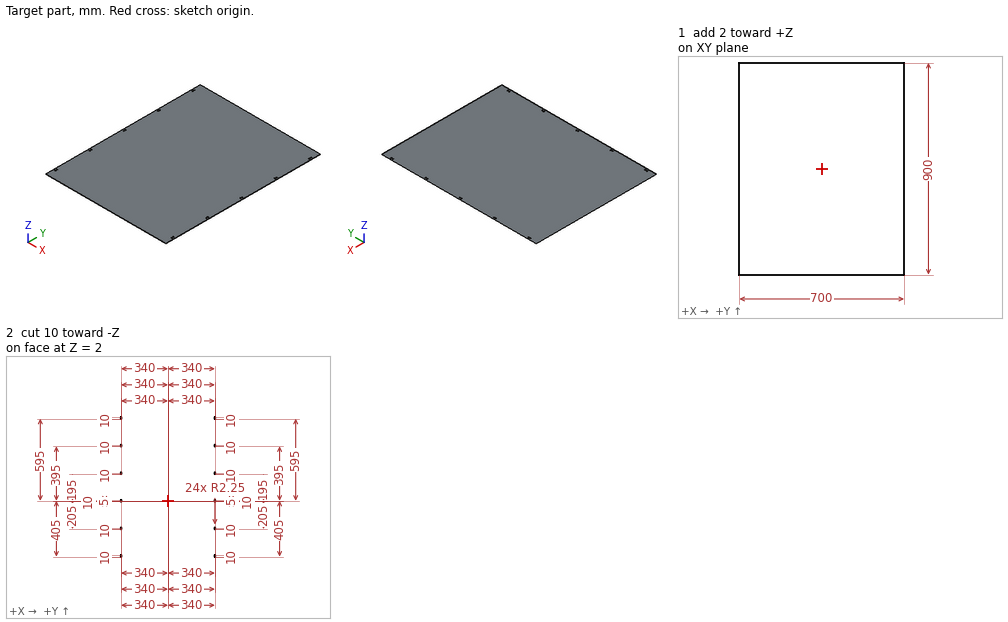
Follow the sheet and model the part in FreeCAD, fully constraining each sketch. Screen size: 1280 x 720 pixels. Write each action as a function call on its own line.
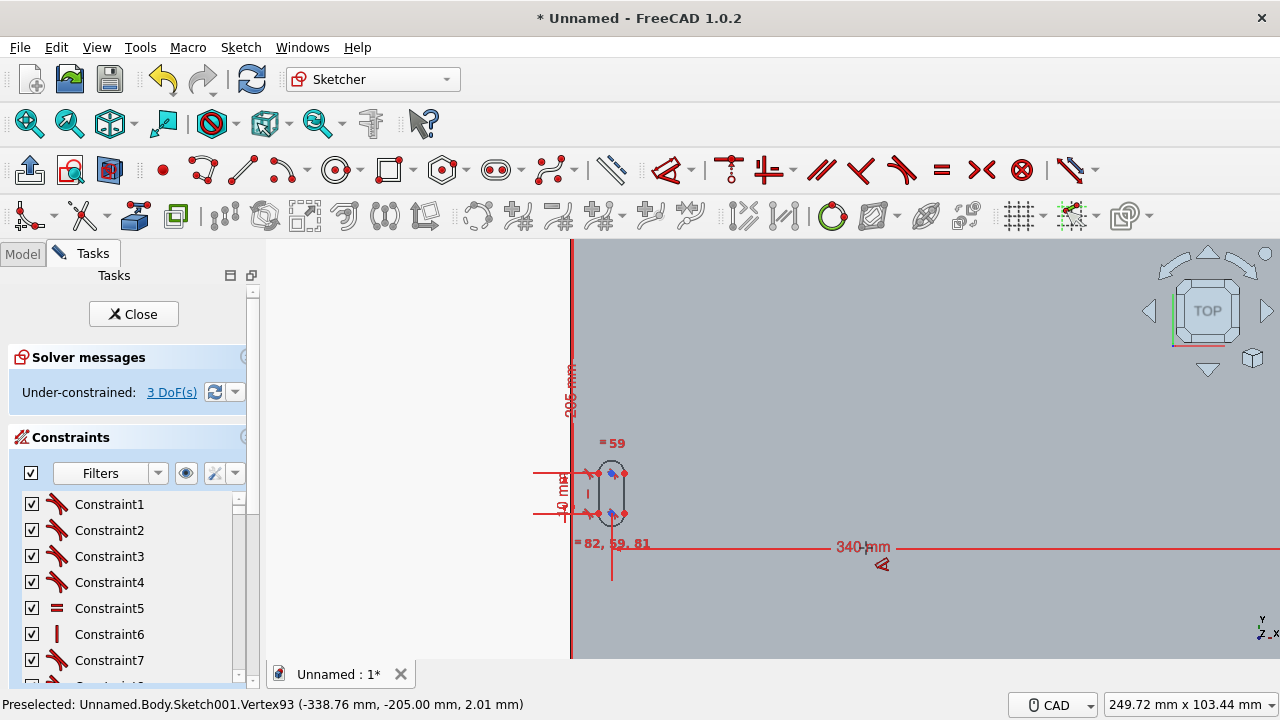
scroll(621, 525, down, 14)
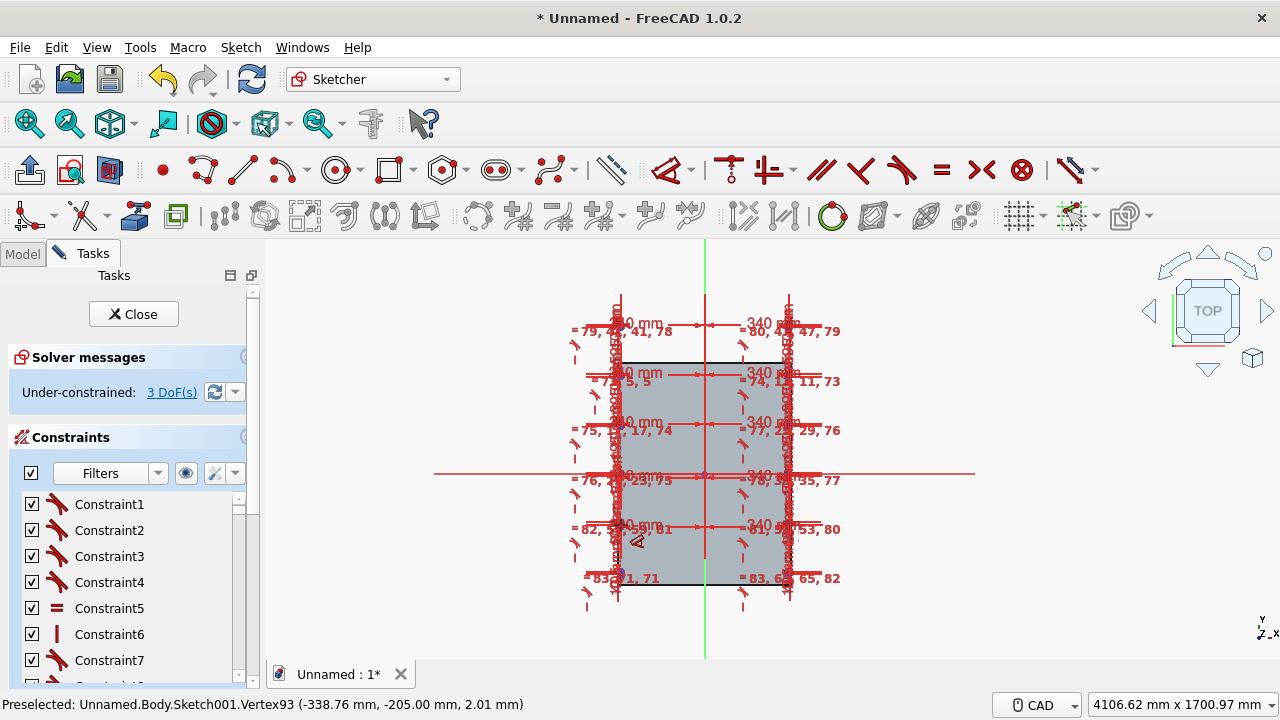
scroll(789, 574, up, 14)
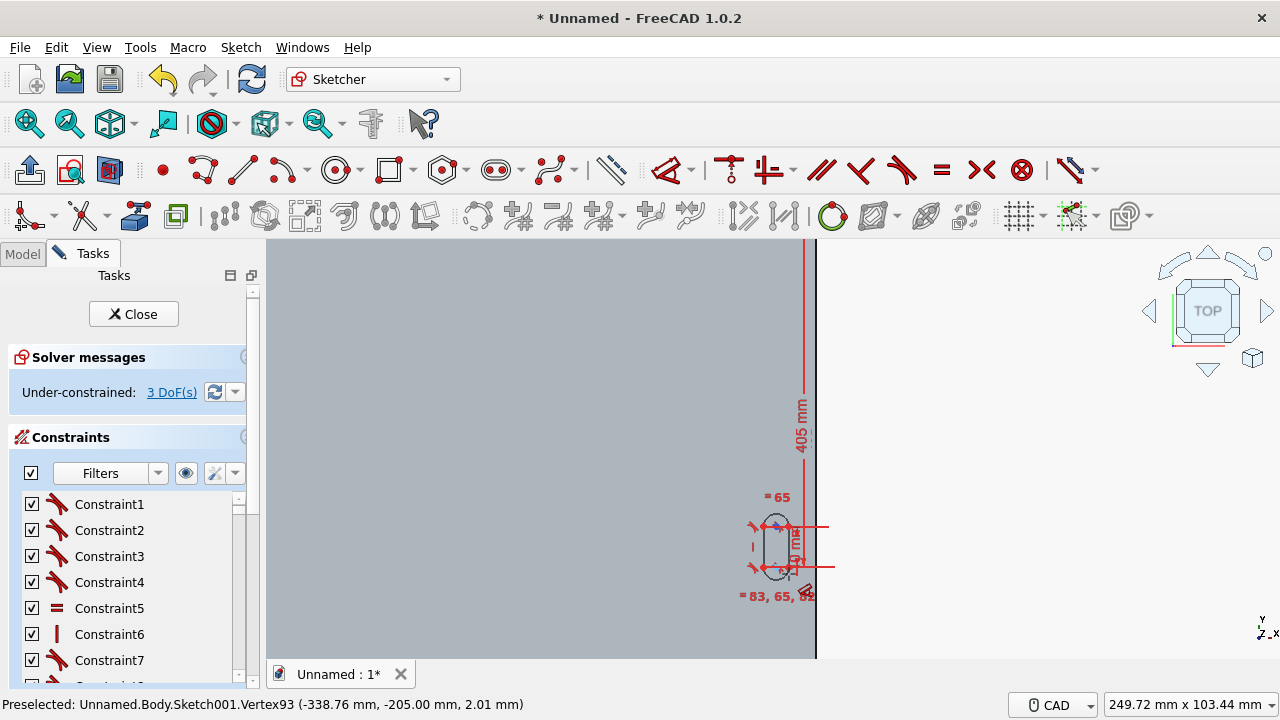
click(776, 567)
click(535, 601)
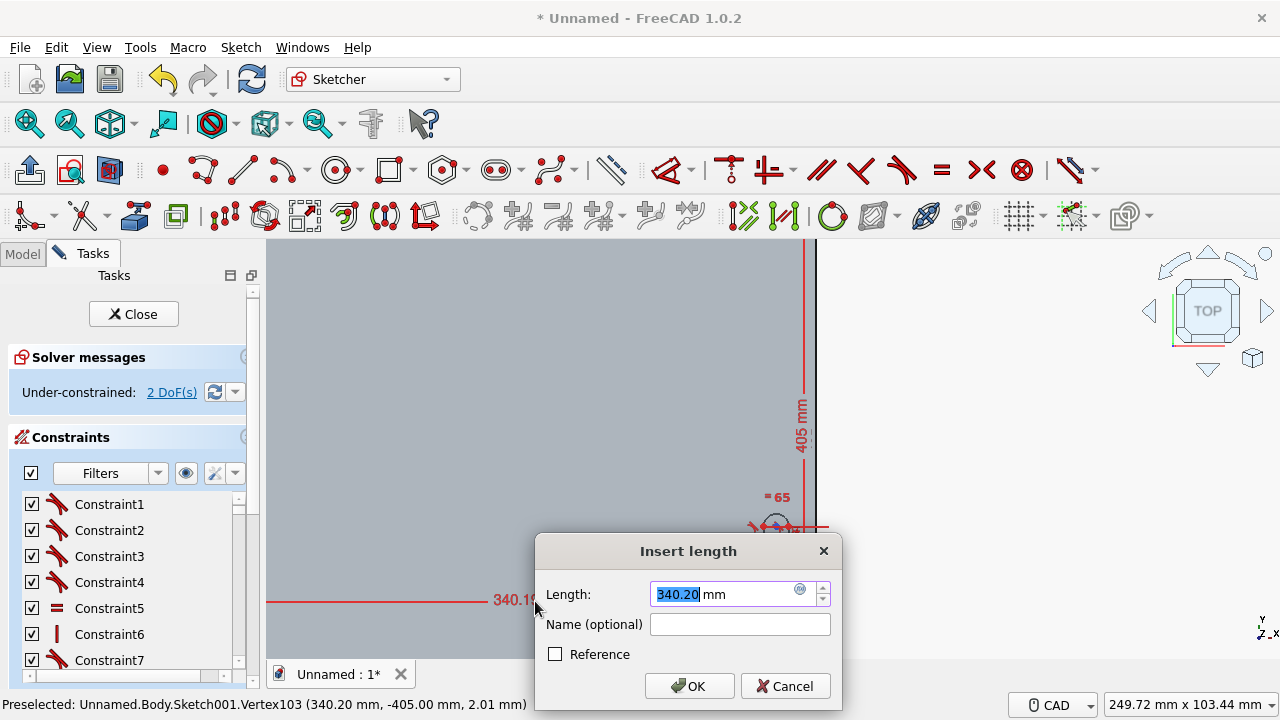
text(340)
key(Return)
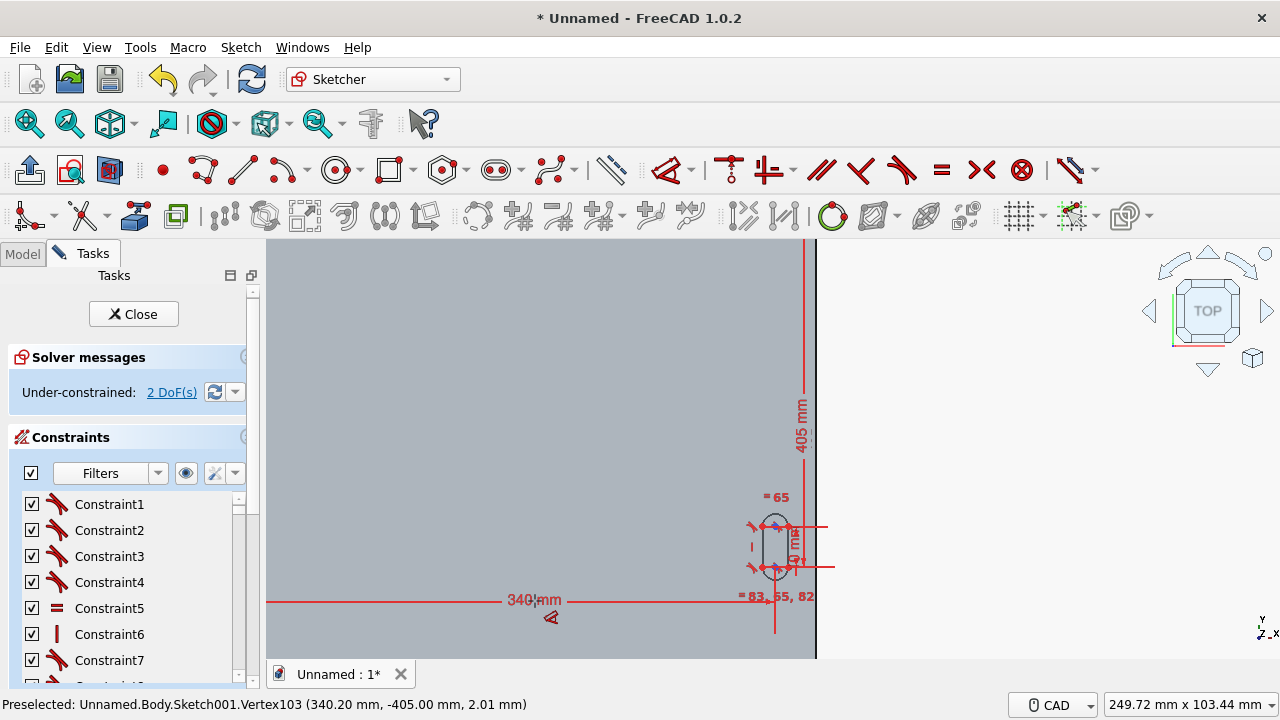
scroll(789, 574, down, 14)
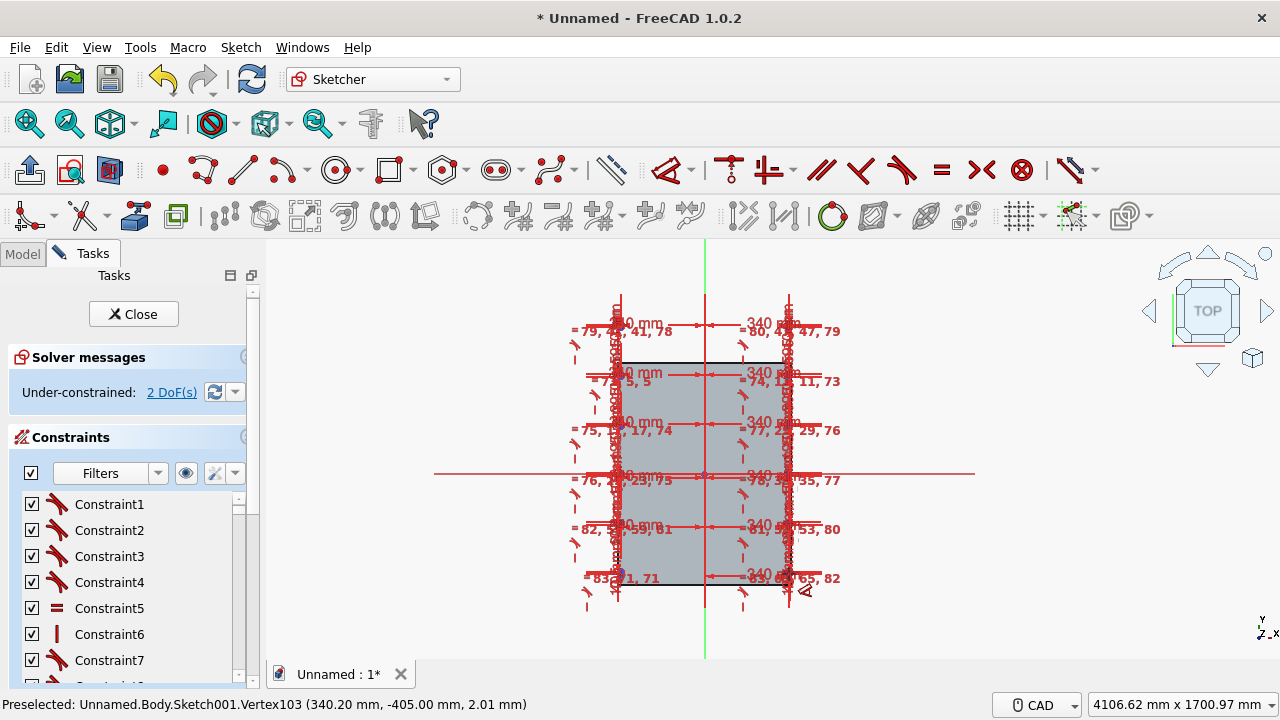
scroll(621, 574, up, 14)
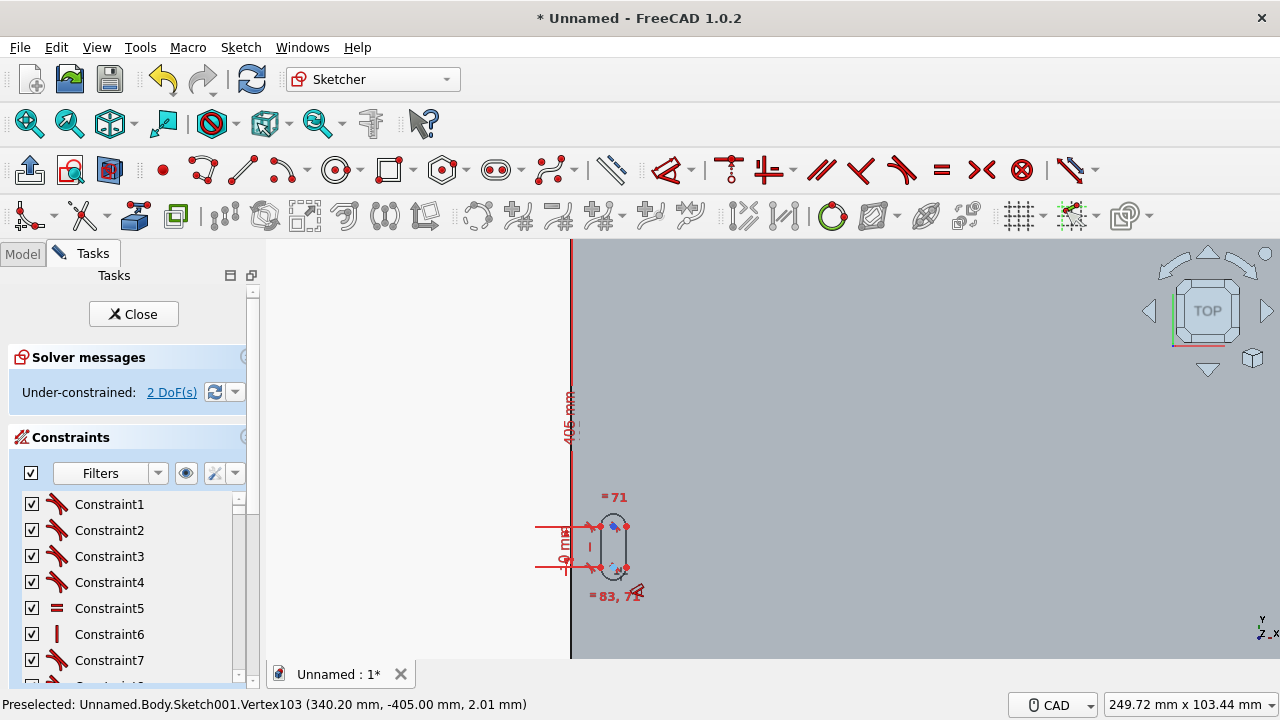
click(613, 567)
click(864, 601)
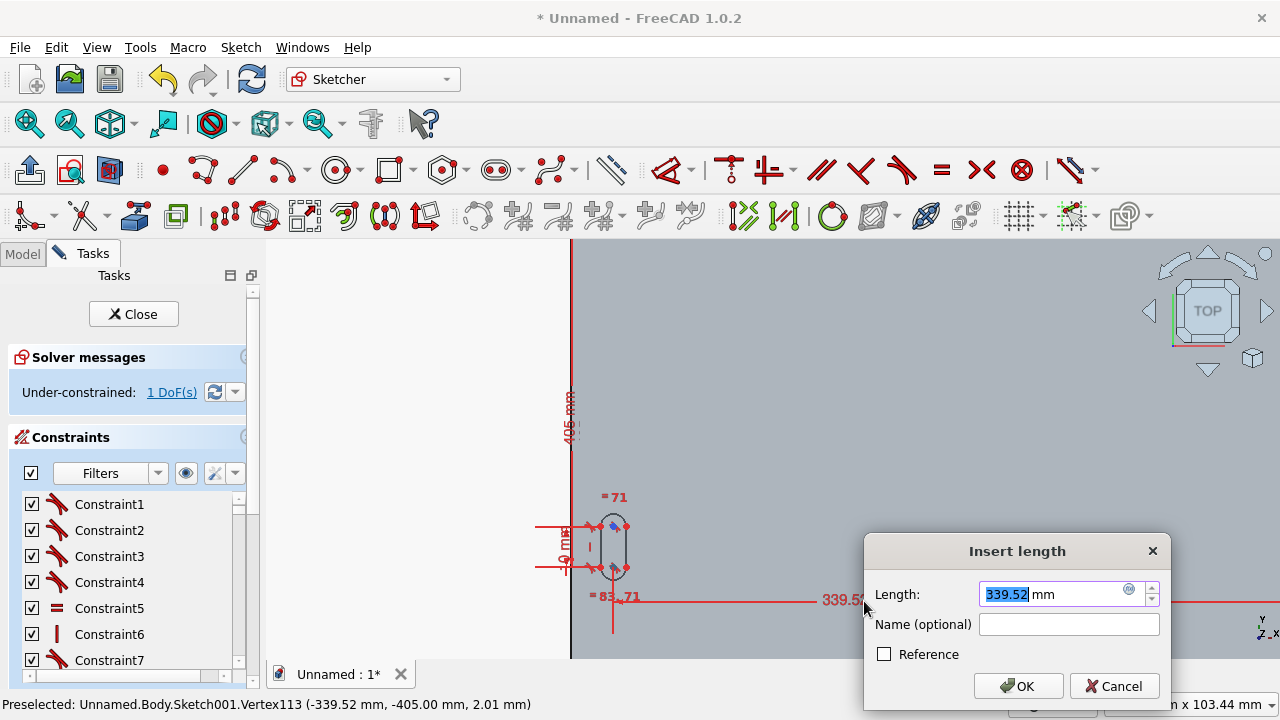
text(340)
key(Return)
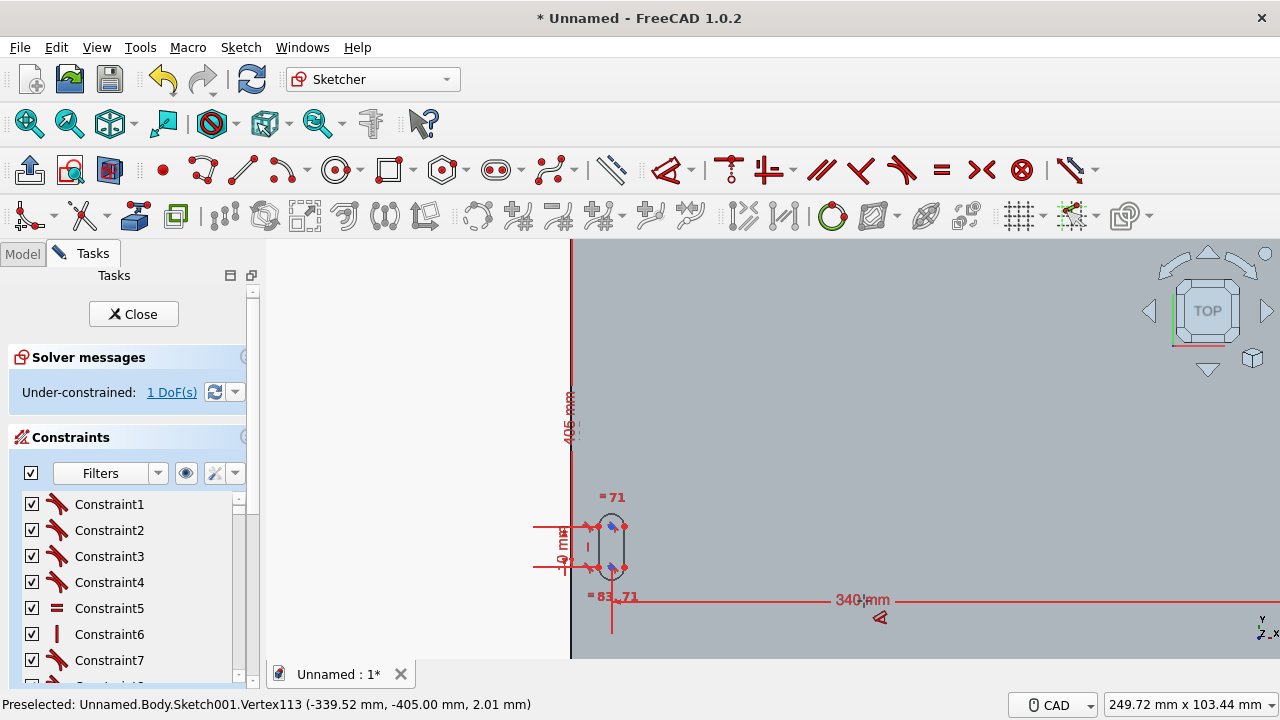
scroll(621, 574, down, 14)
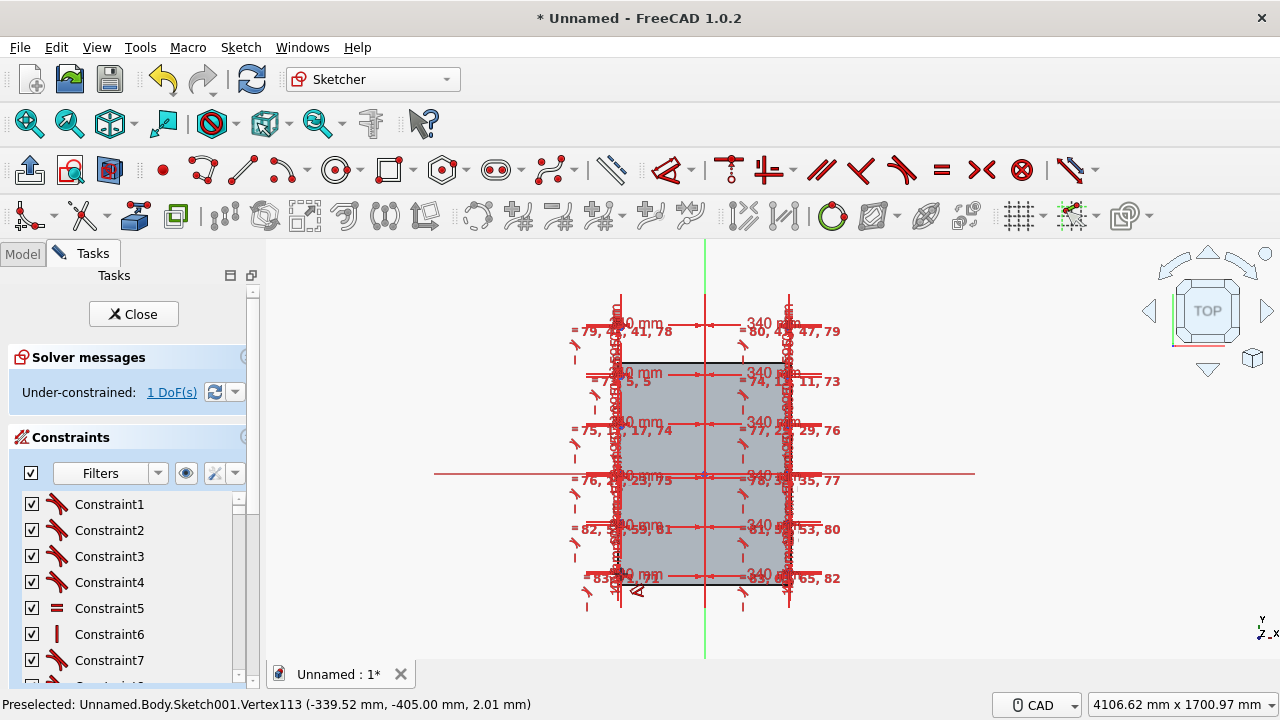
scroll(620, 377, up, 22)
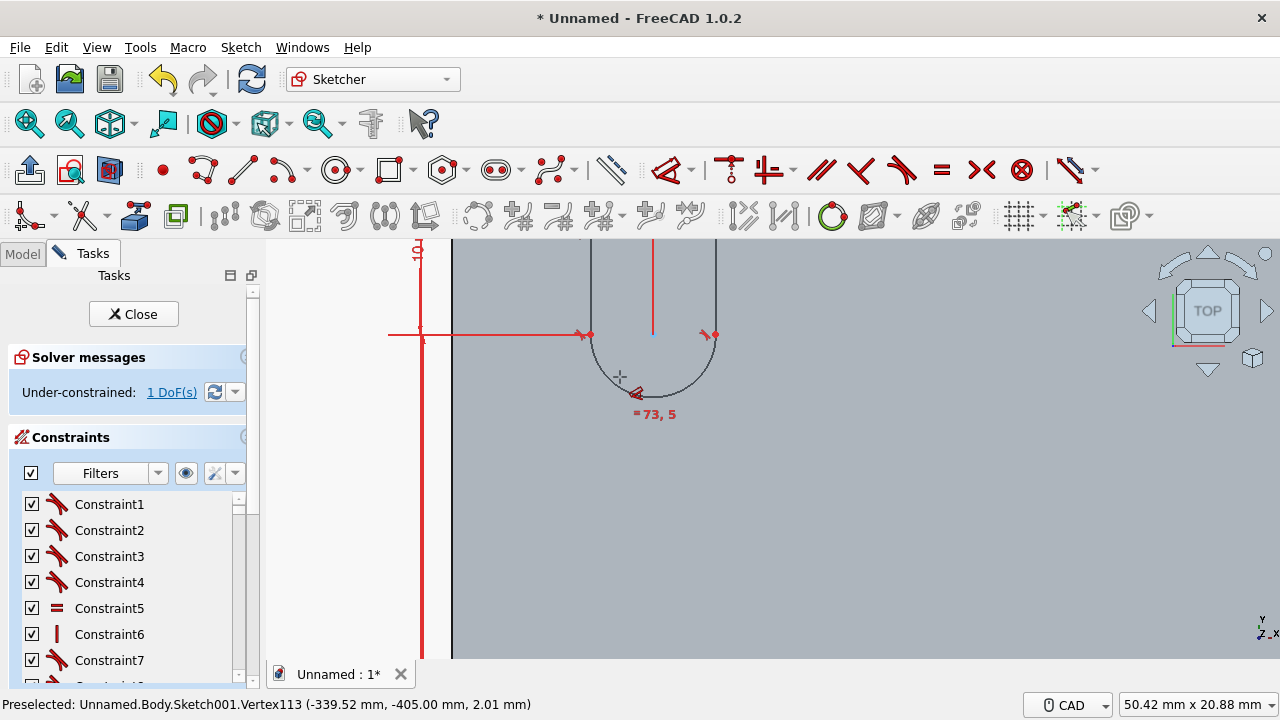
click(617, 385)
click(598, 411)